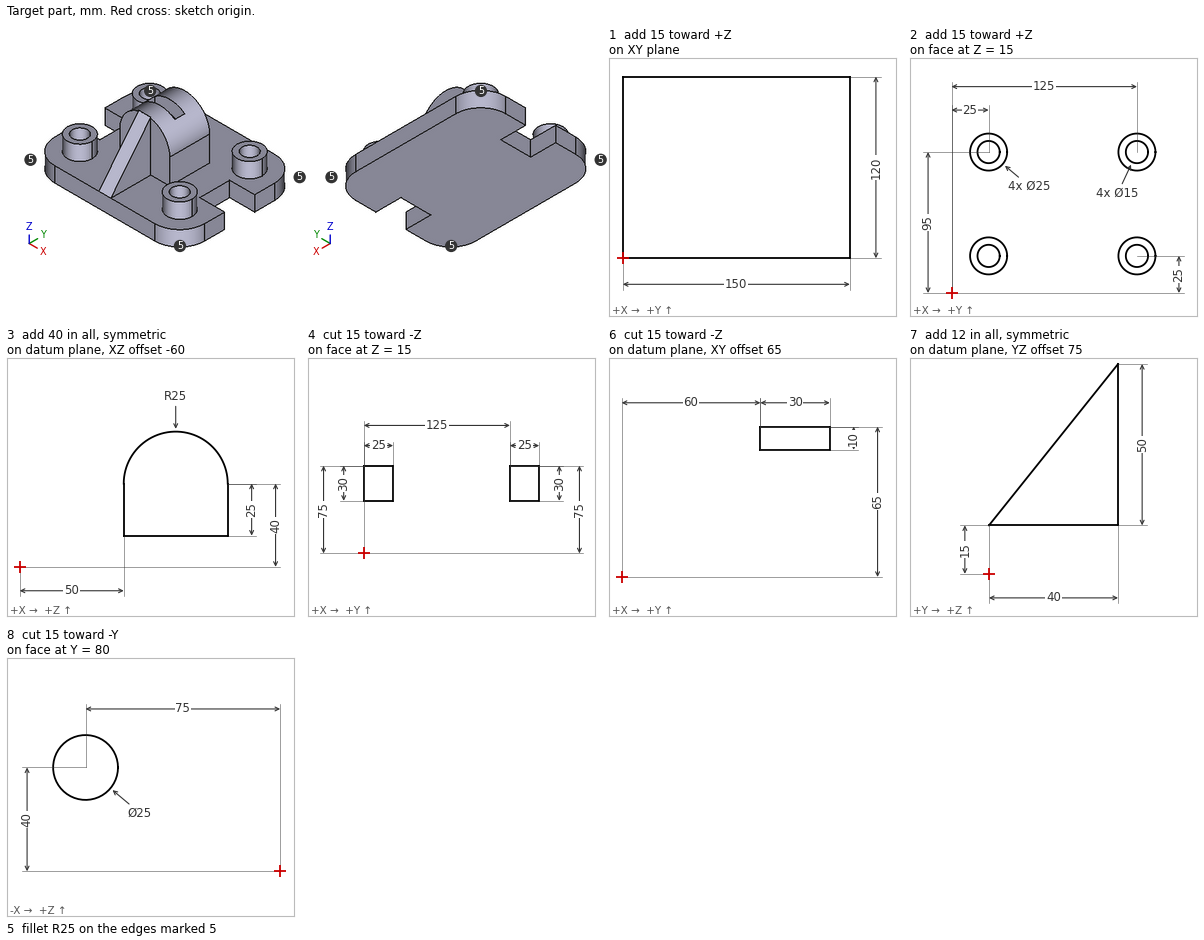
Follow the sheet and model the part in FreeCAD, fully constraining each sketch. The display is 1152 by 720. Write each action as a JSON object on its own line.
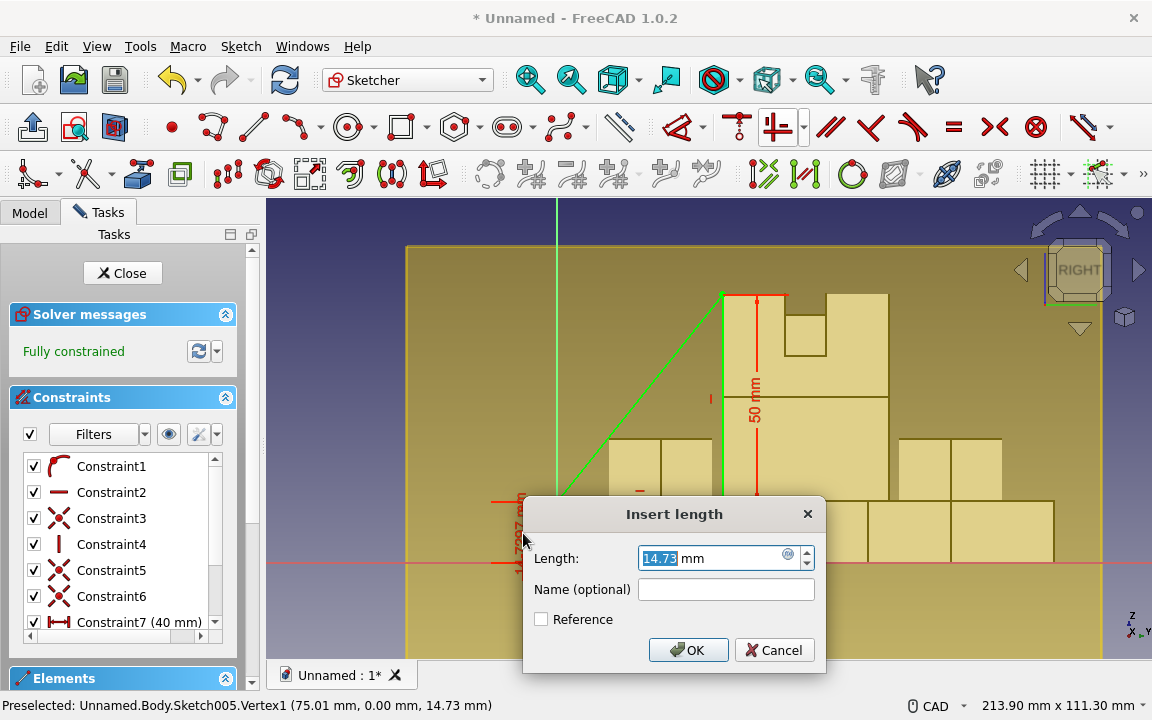
{"action": "type", "text": "15"}
{"action": "key", "text": "Return"}
{"action": "key", "text": "Escape"}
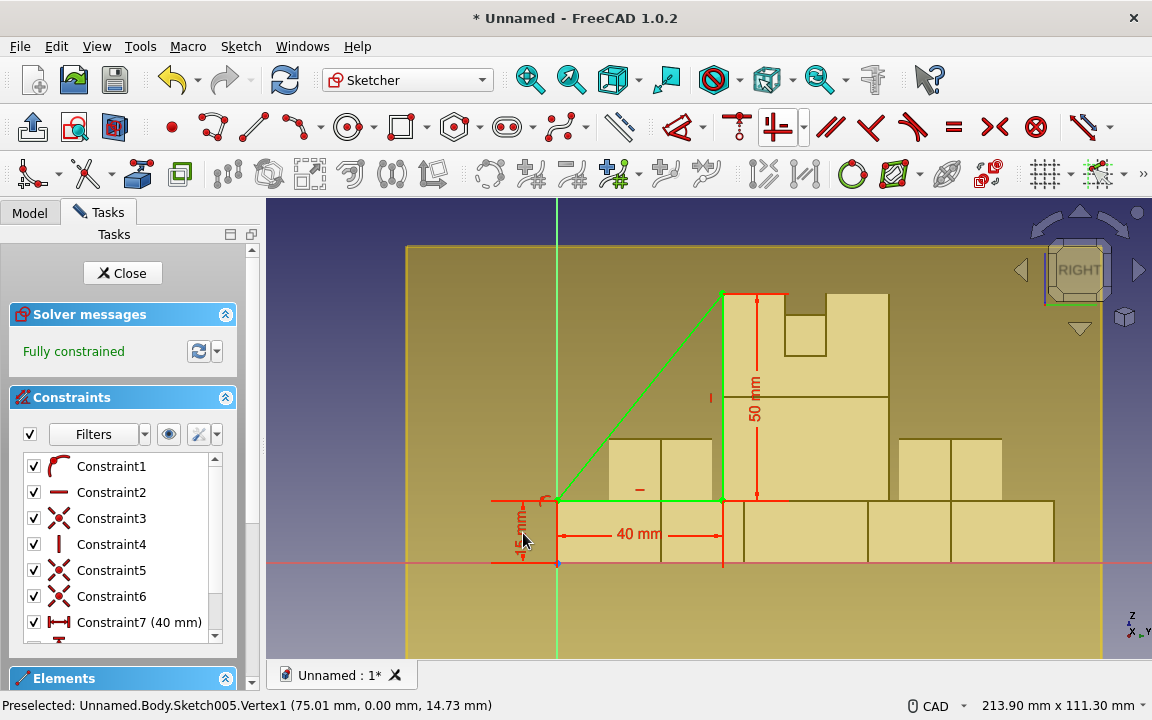
{"action": "left_click", "coordinate": [123, 273]}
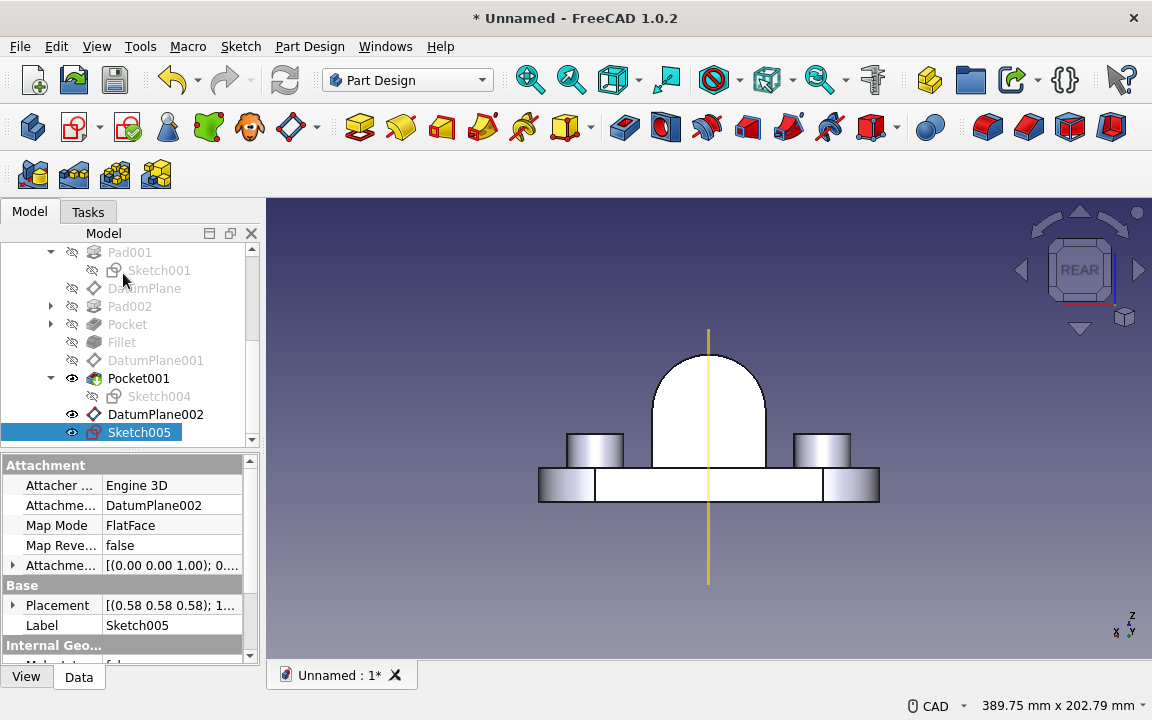
{"action": "left_click", "coordinate": [360, 128]}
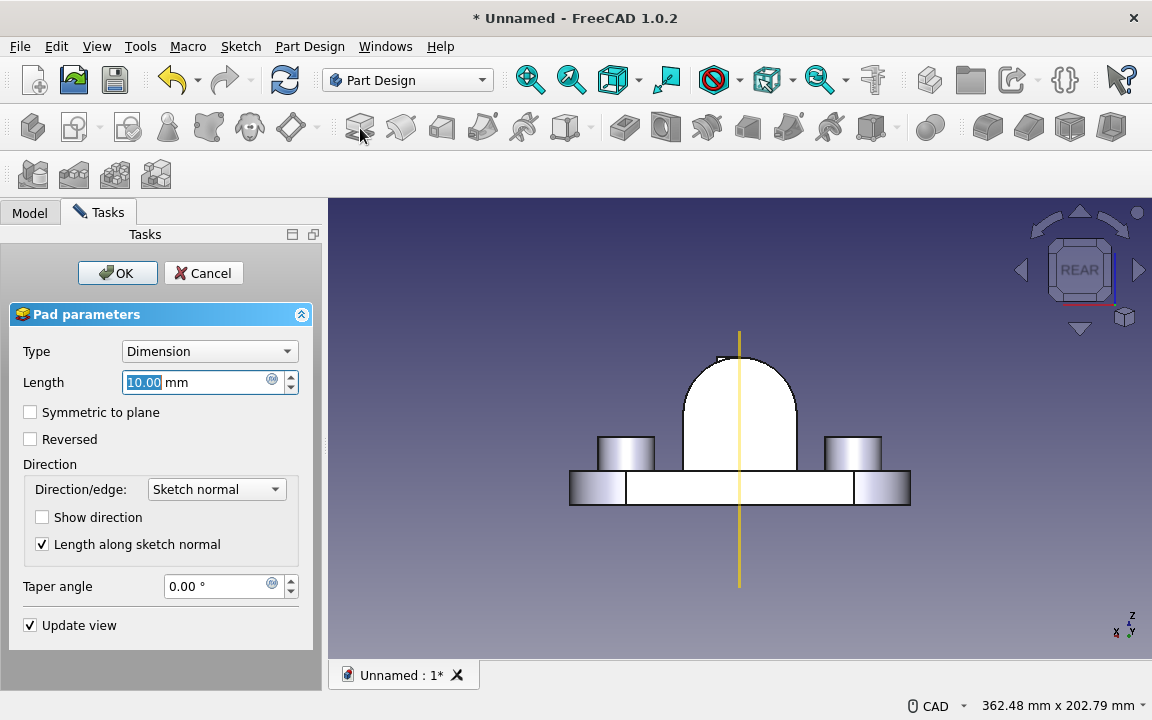
{"action": "type", "text": "12"}
{"action": "key", "text": "Tab"}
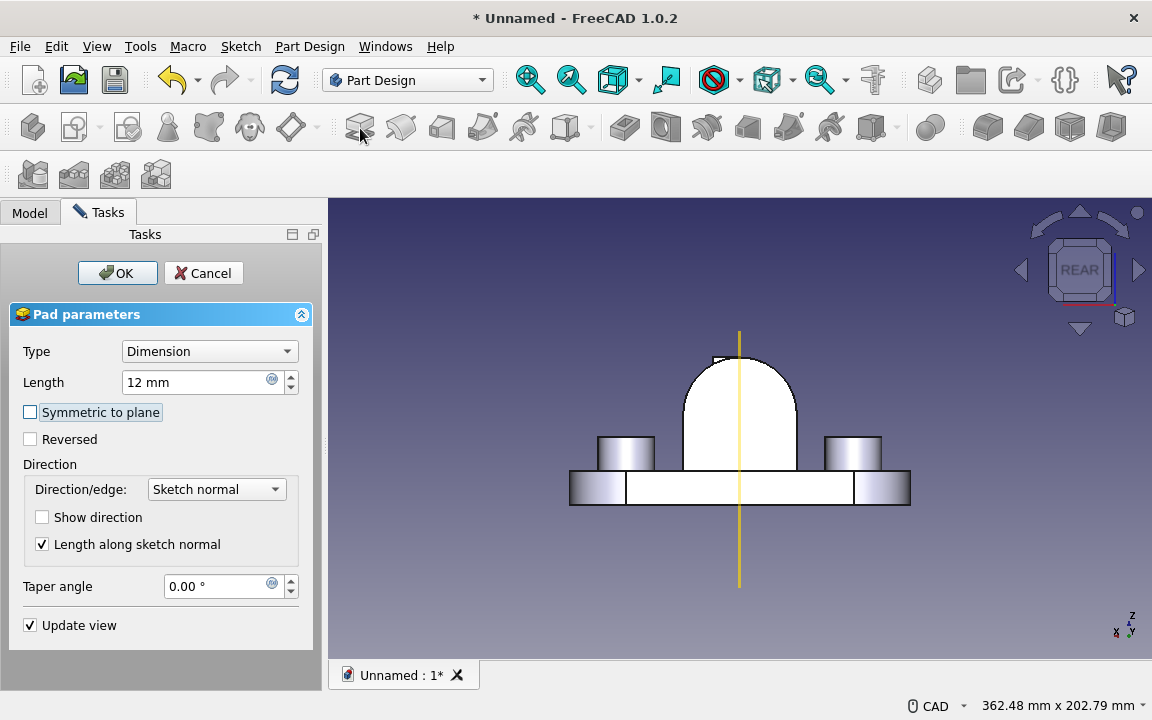
{"action": "left_click", "coordinate": [31, 412]}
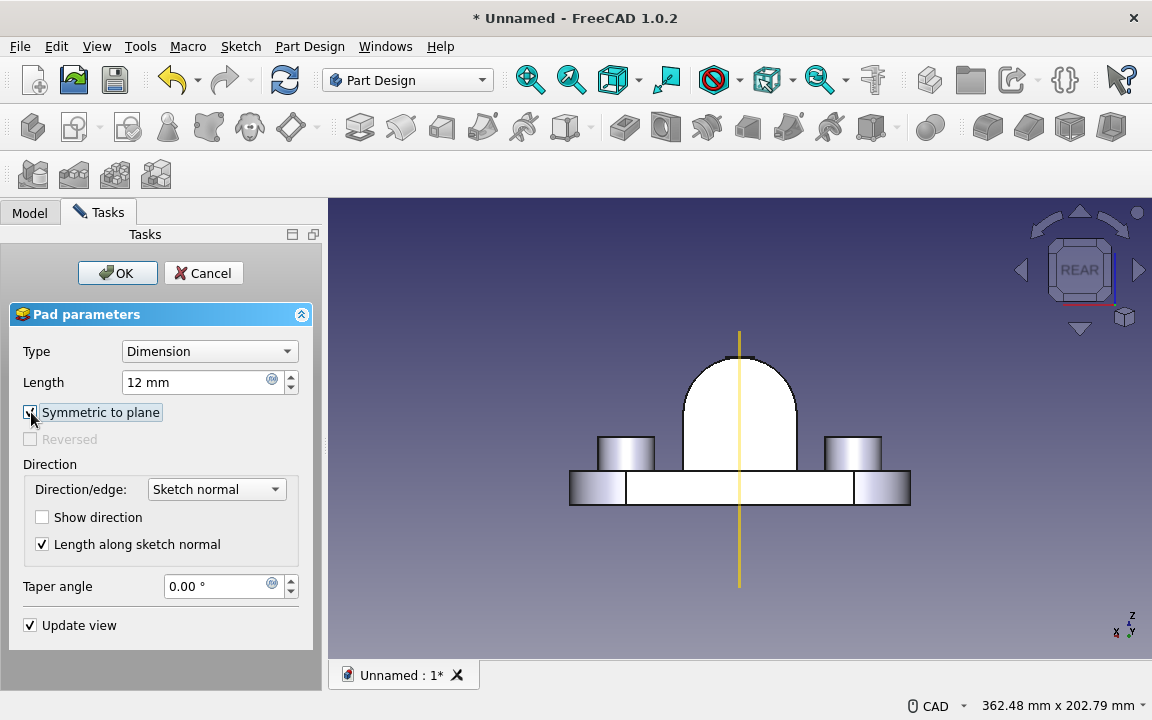
{"action": "left_click", "coordinate": [118, 273]}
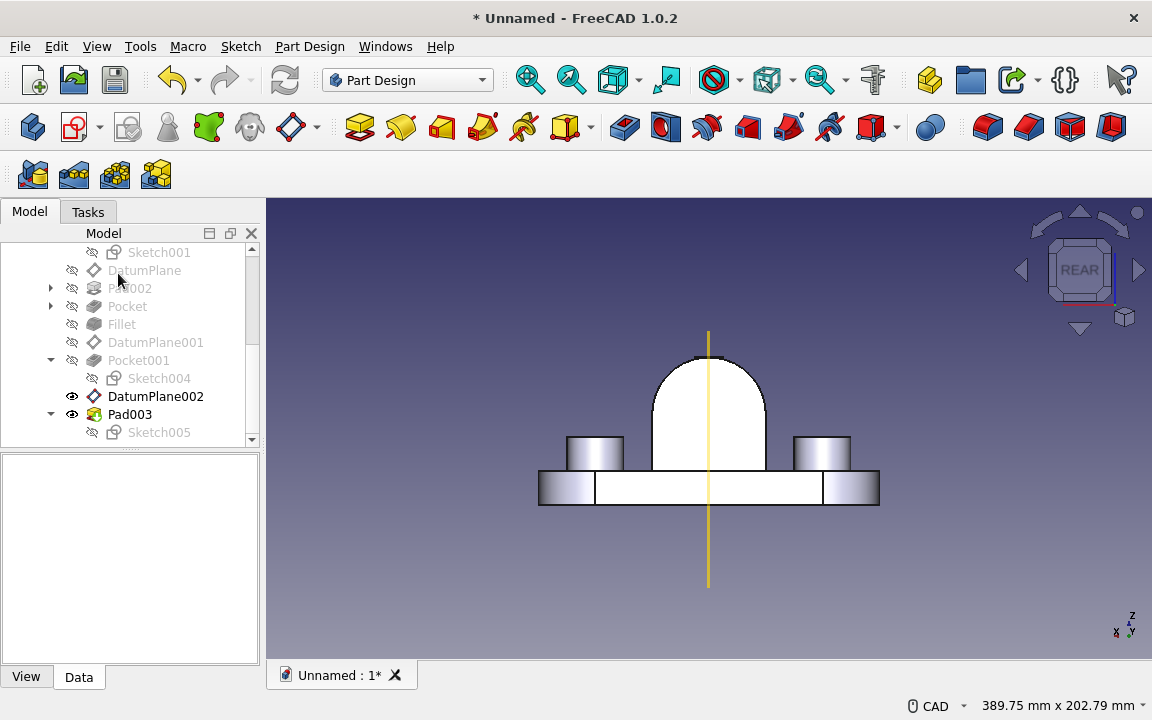
{"action": "left_click", "coordinate": [117, 396]}
{"action": "key", "text": "space"}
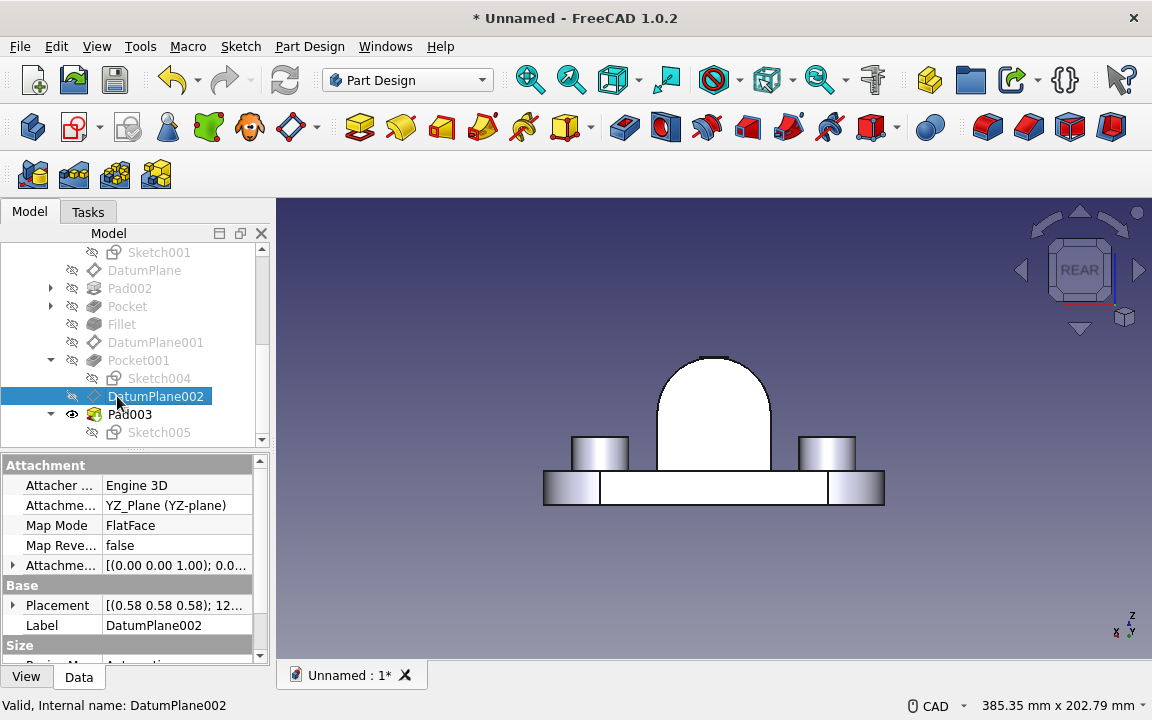
{"action": "left_click", "coordinate": [531, 80]}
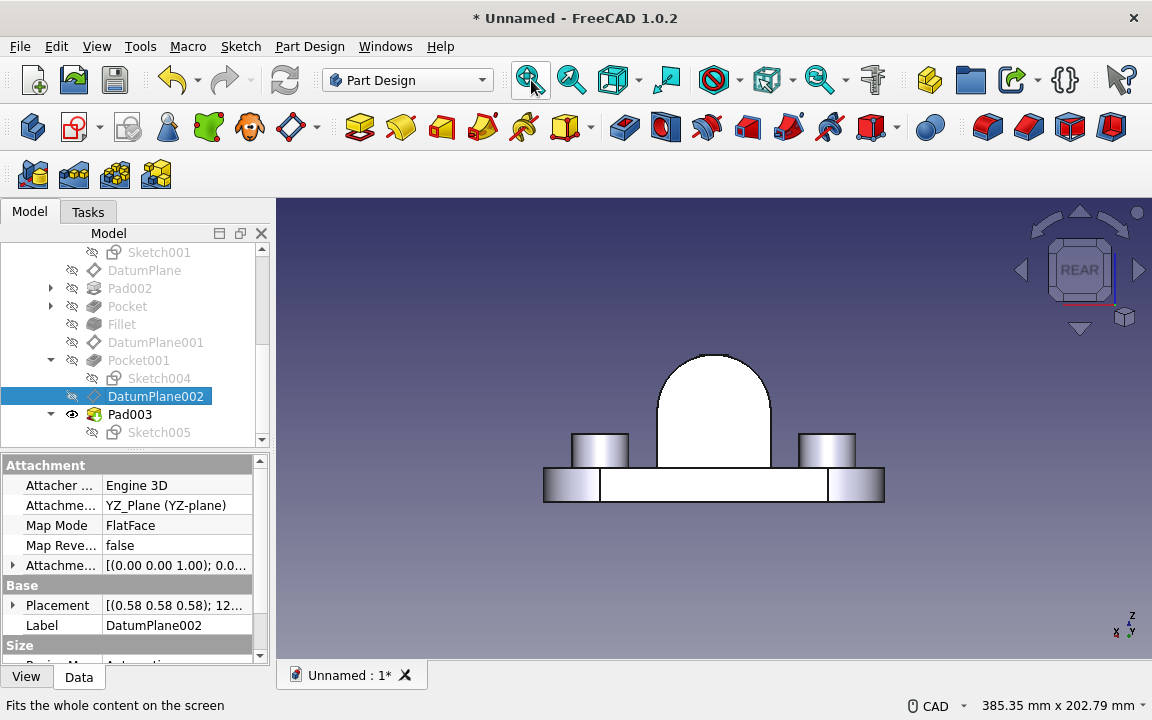
{"action": "left_click", "coordinate": [714, 410]}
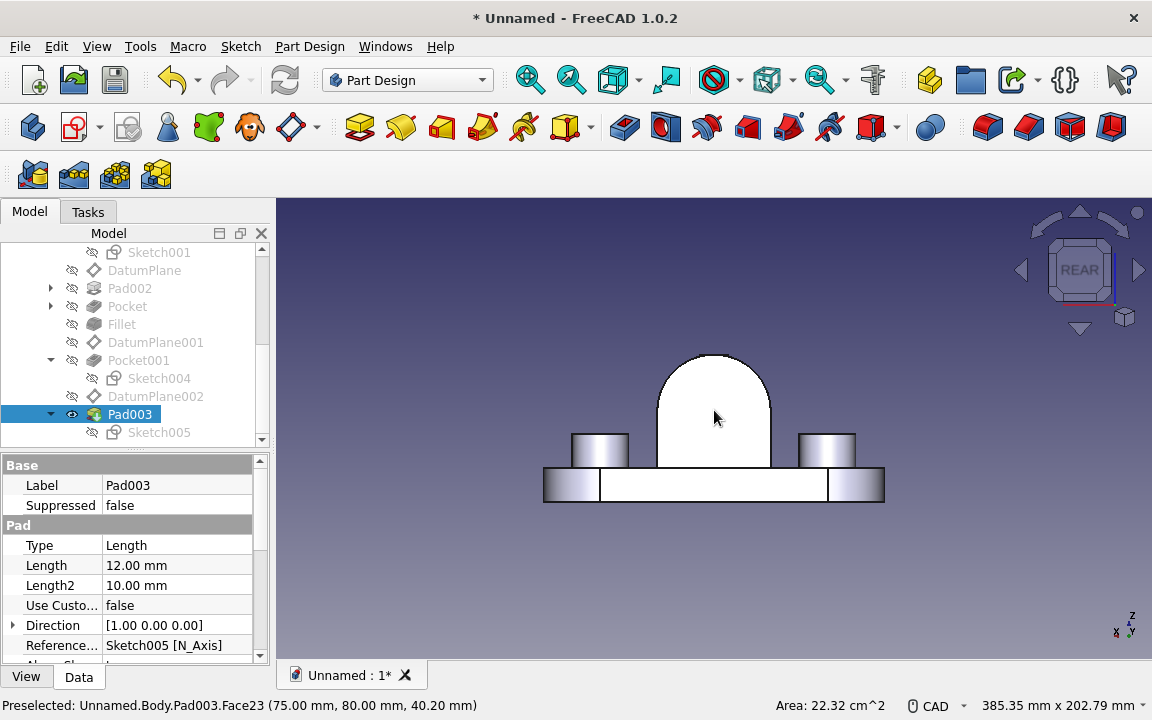
{"action": "left_click", "coordinate": [74, 128]}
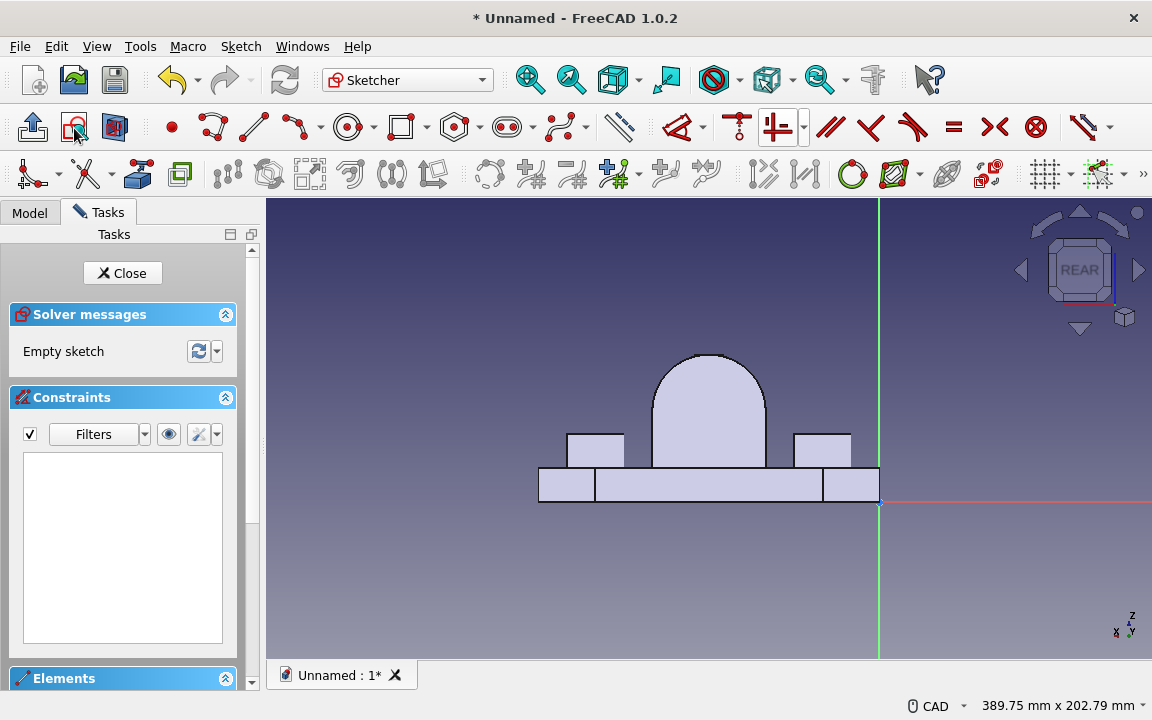
{"action": "scroll", "coordinate": [726, 407], "scroll_direction": "up", "scroll_amount": 8}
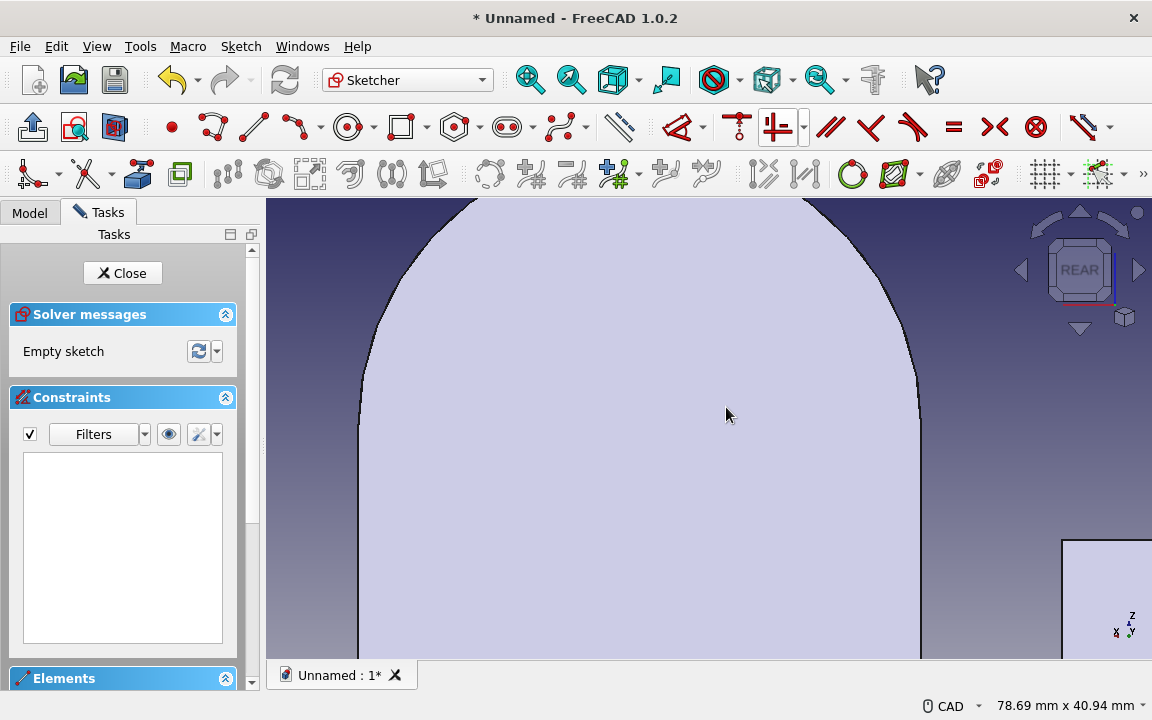
{"action": "key", "text": "g c"}